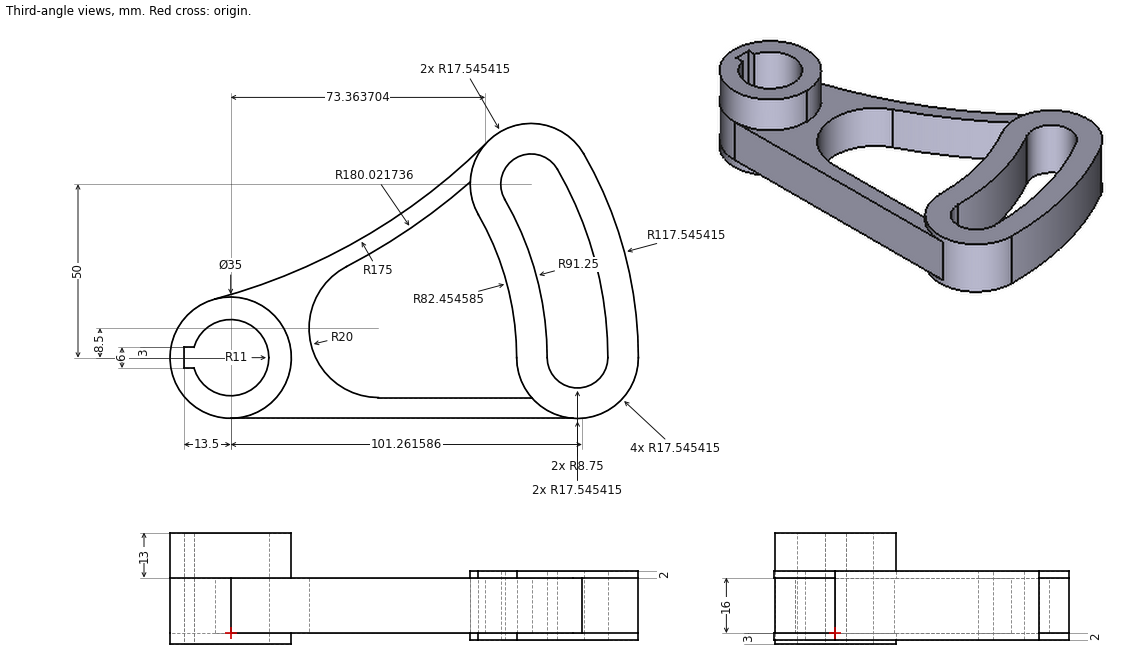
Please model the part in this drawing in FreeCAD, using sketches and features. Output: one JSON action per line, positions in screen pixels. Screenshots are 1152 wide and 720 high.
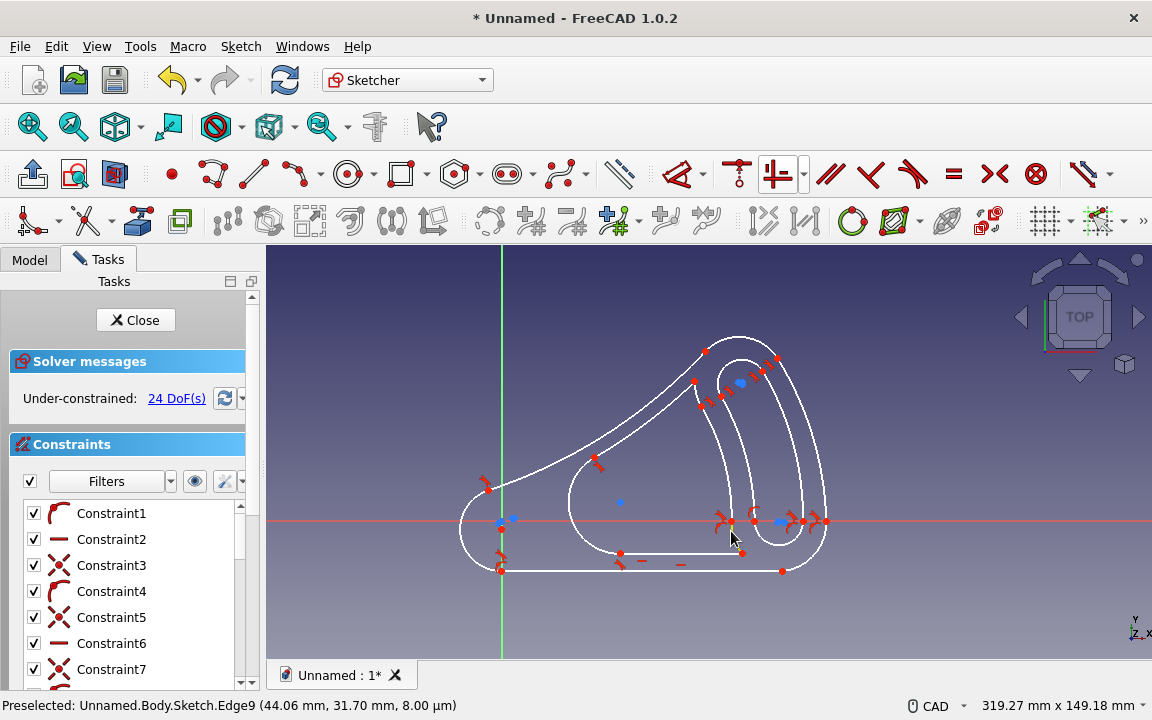
{"action": "left_click", "coordinate": [759, 342]}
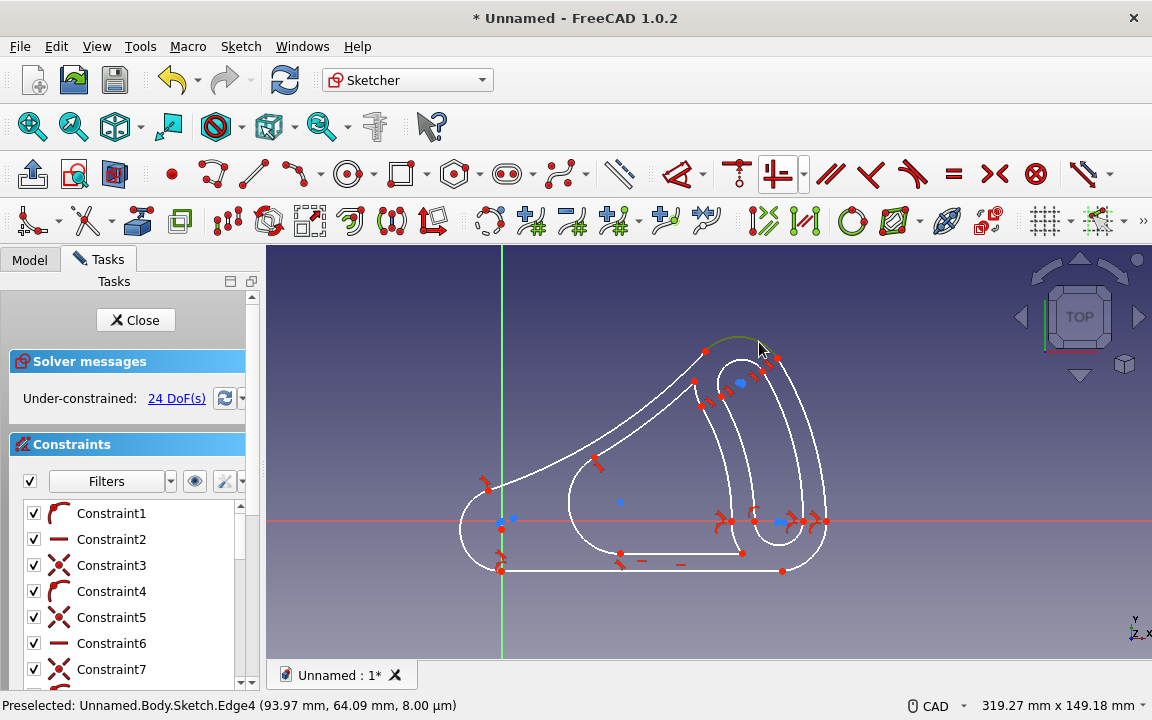
{"action": "scroll", "coordinate": [696, 395], "scroll_direction": "up", "scroll_amount": 2}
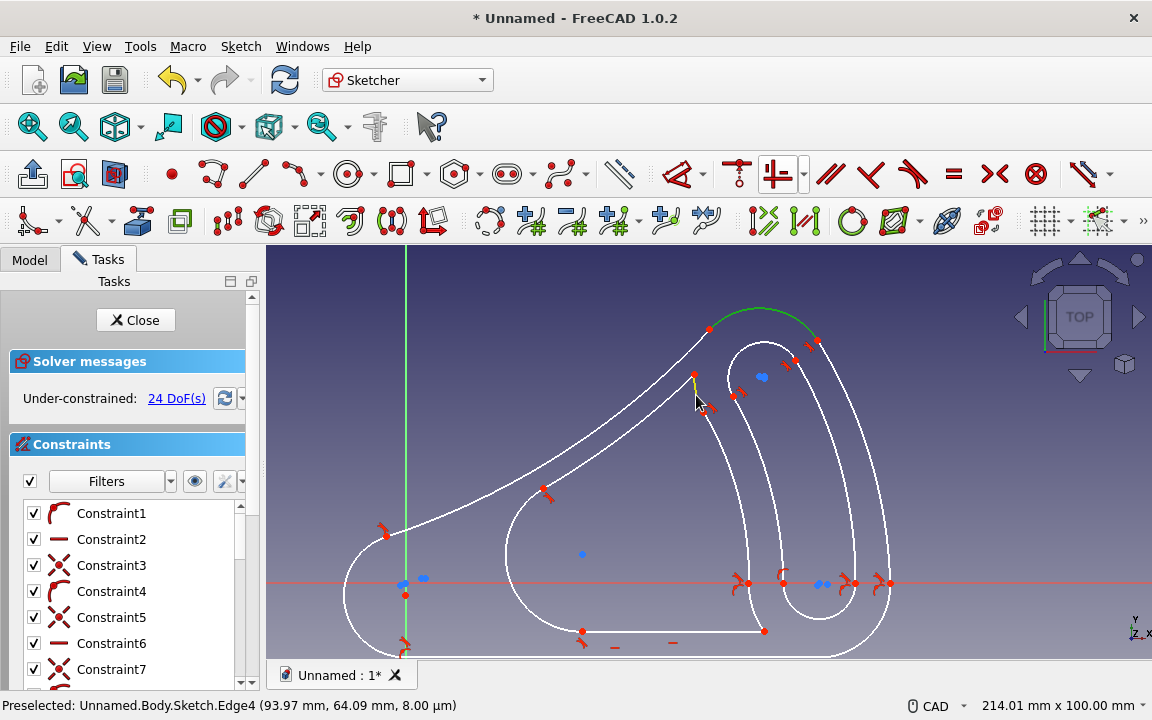
{"action": "left_click", "coordinate": [696, 394]}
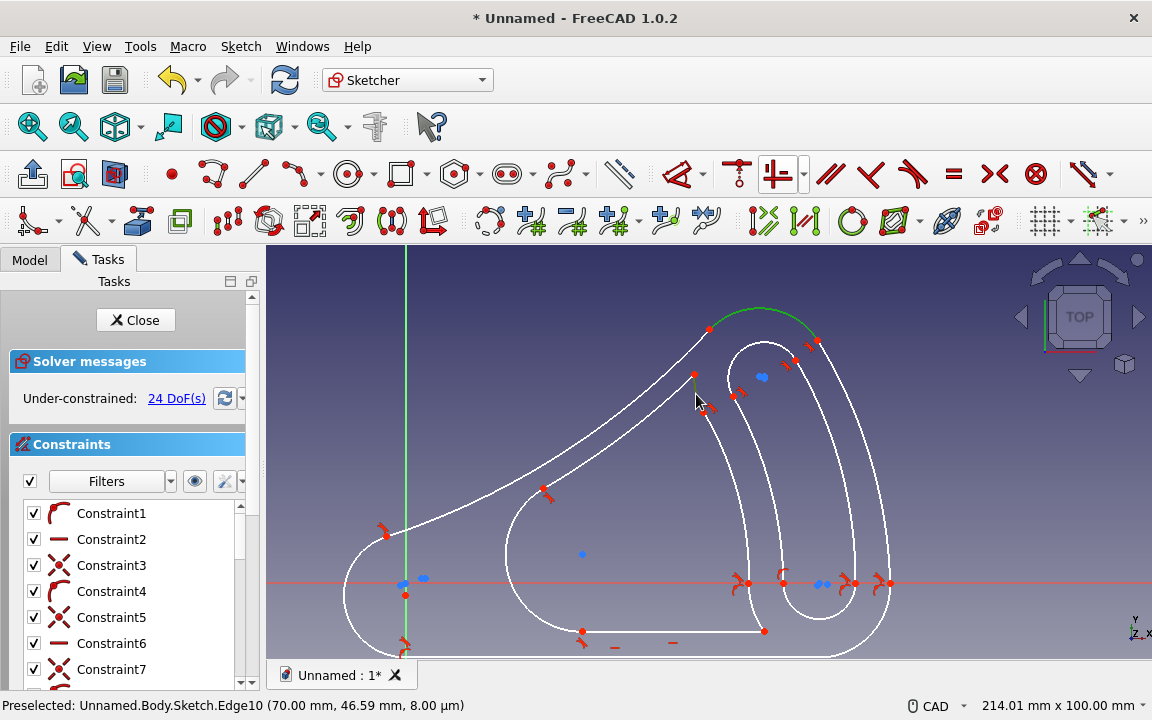
{"action": "left_click", "coordinate": [737, 174]}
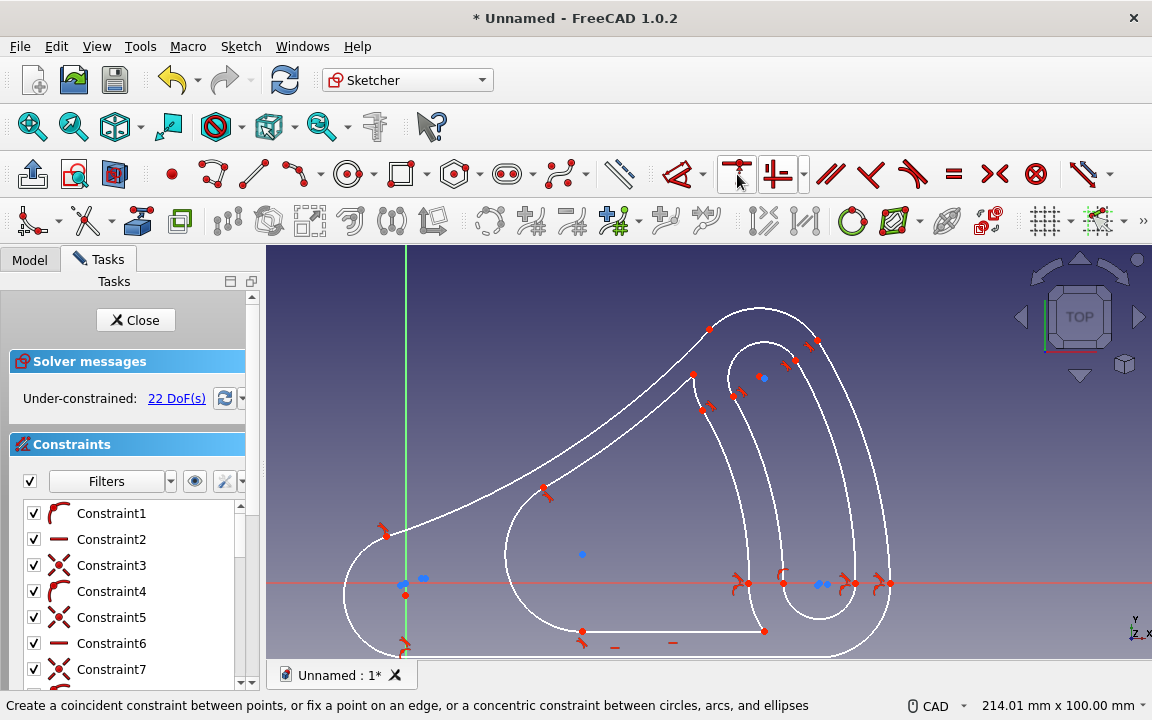
{"action": "left_click", "coordinate": [882, 507]}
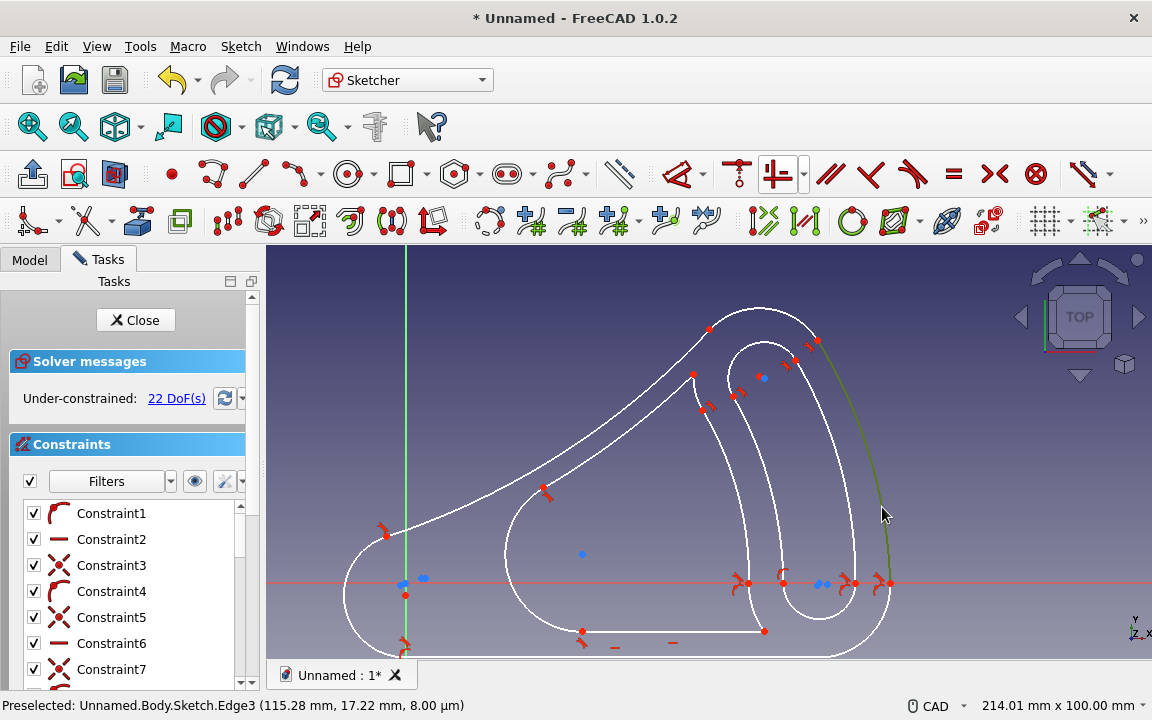
{"action": "left_click", "coordinate": [745, 529]}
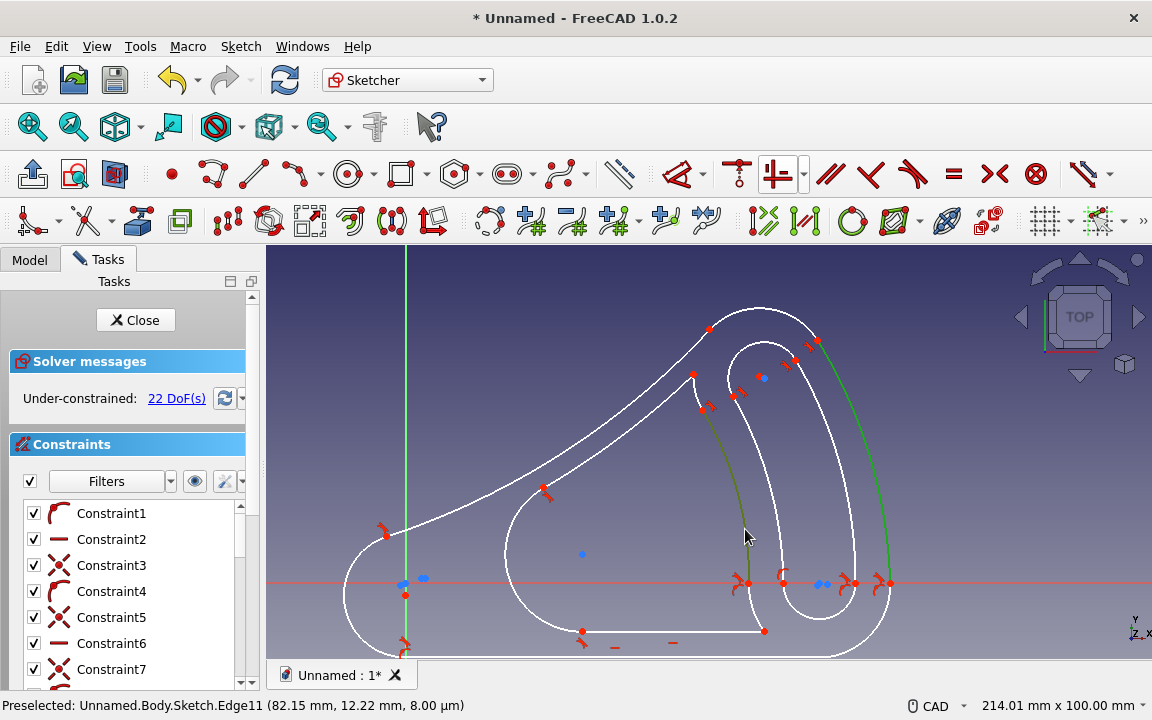
{"action": "left_click", "coordinate": [737, 174]}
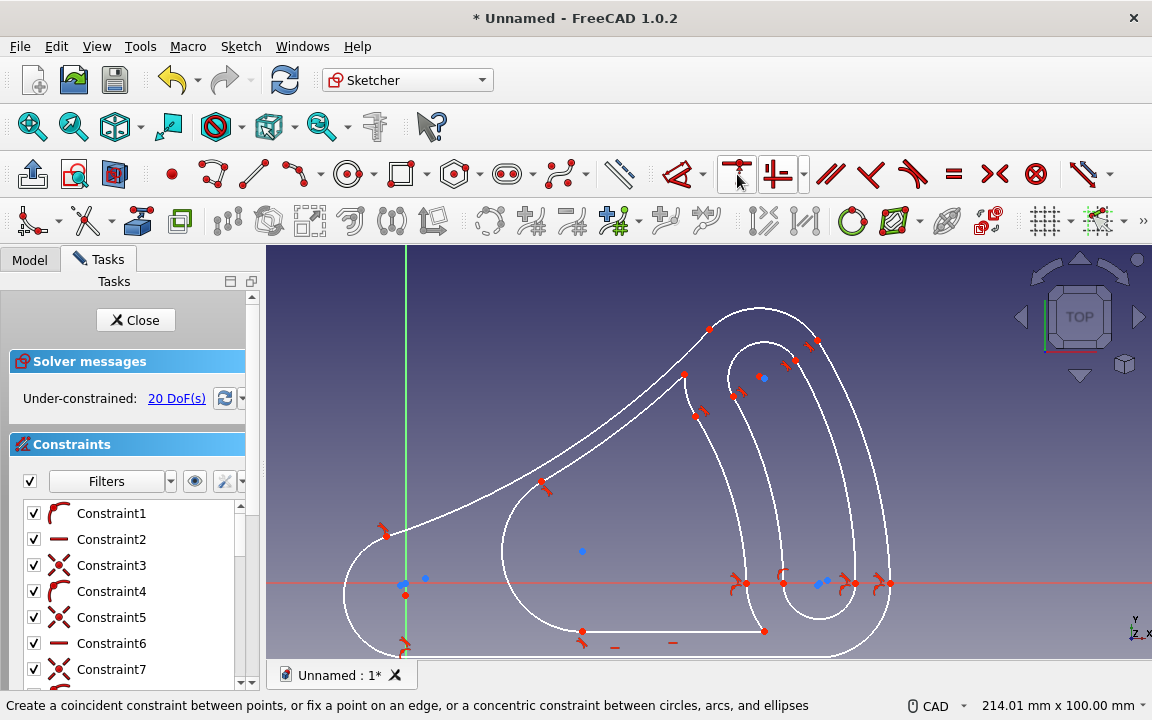
{"action": "left_click", "coordinate": [790, 316]}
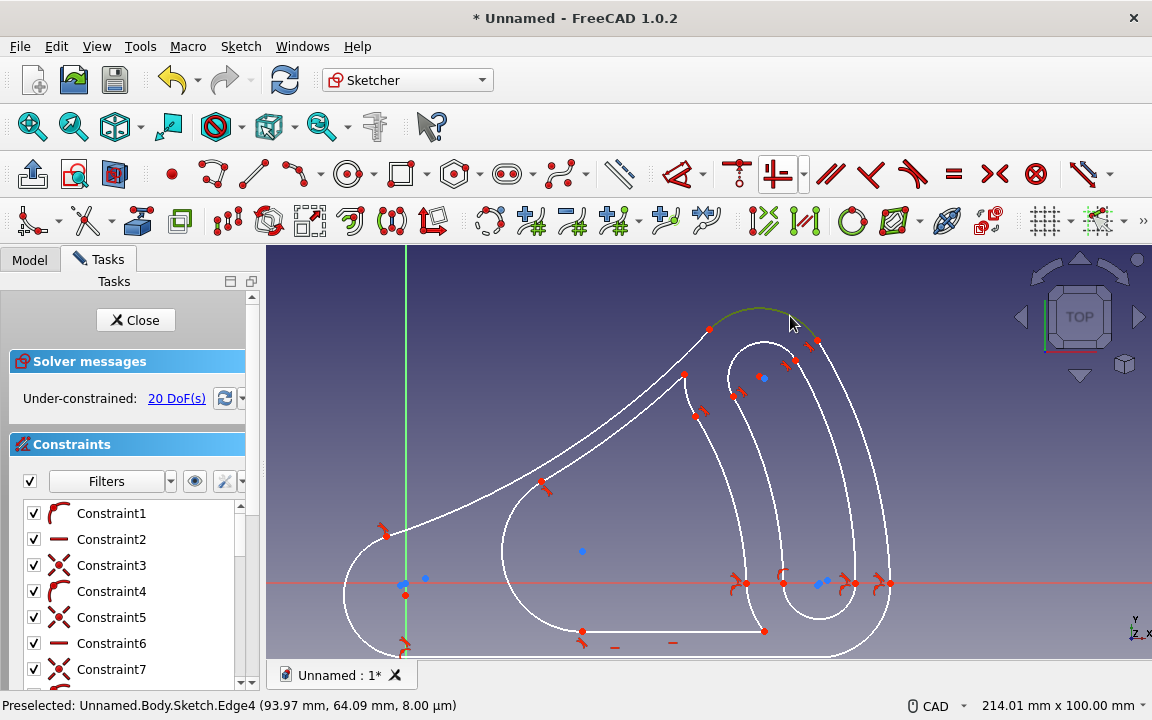
{"action": "left_click", "coordinate": [768, 342]}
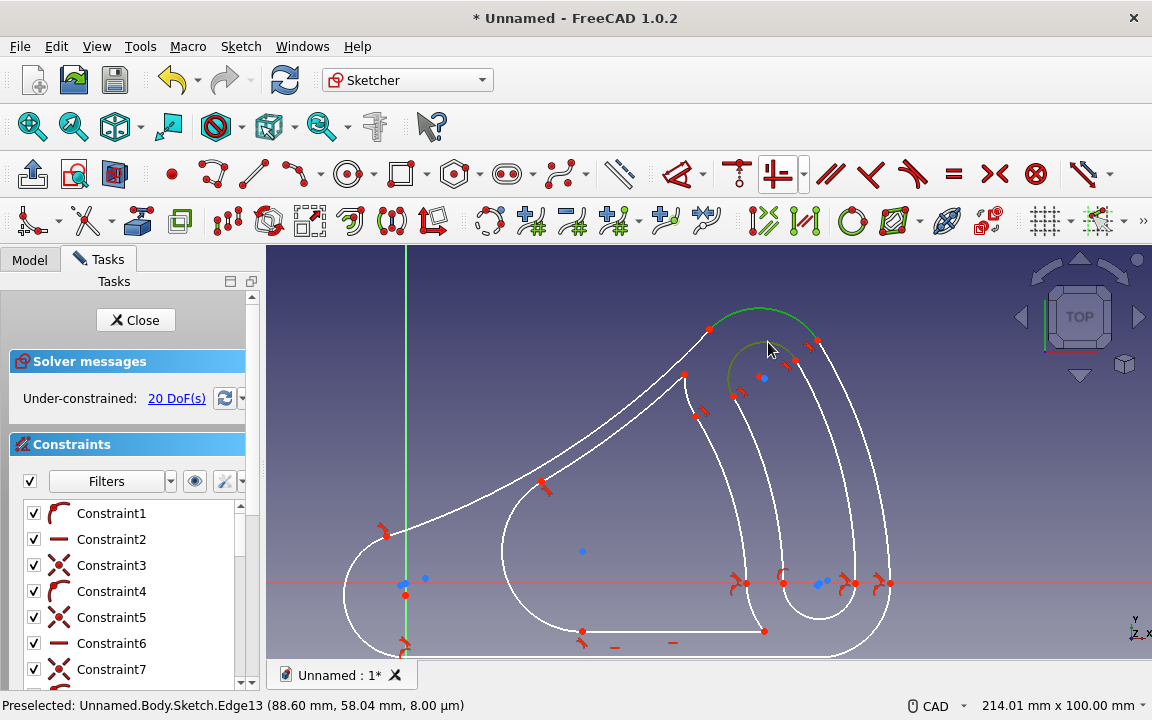
{"action": "left_click", "coordinate": [737, 174]}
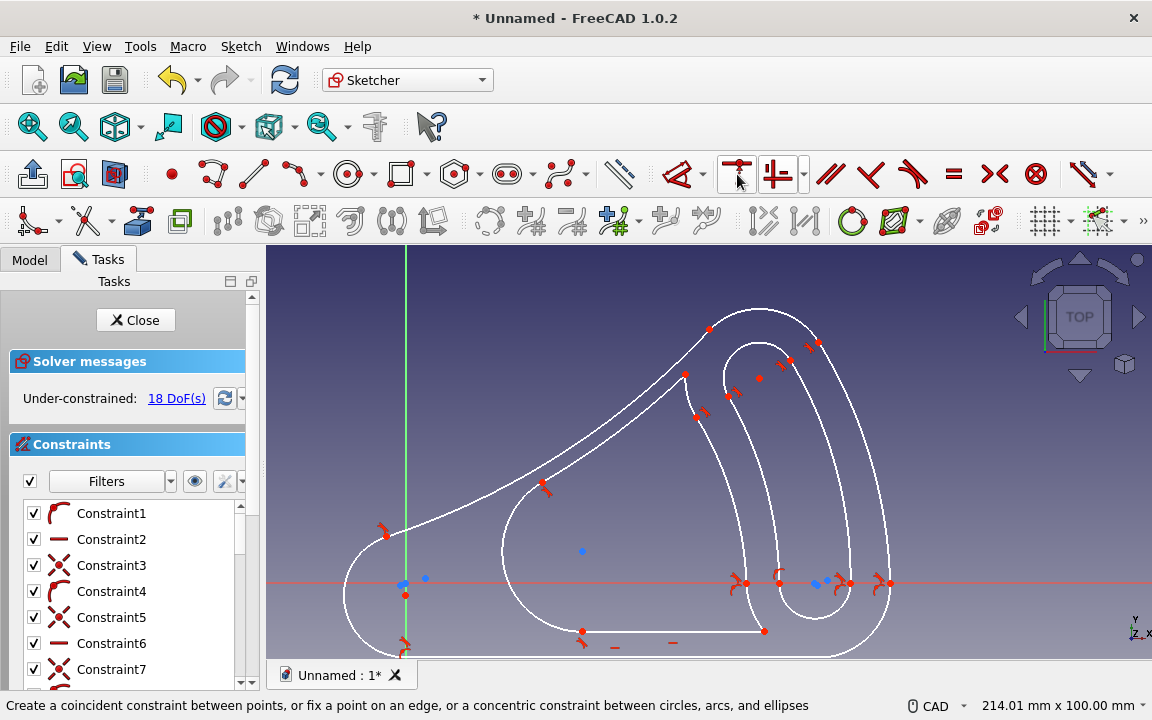
{"action": "left_click", "coordinate": [882, 508]}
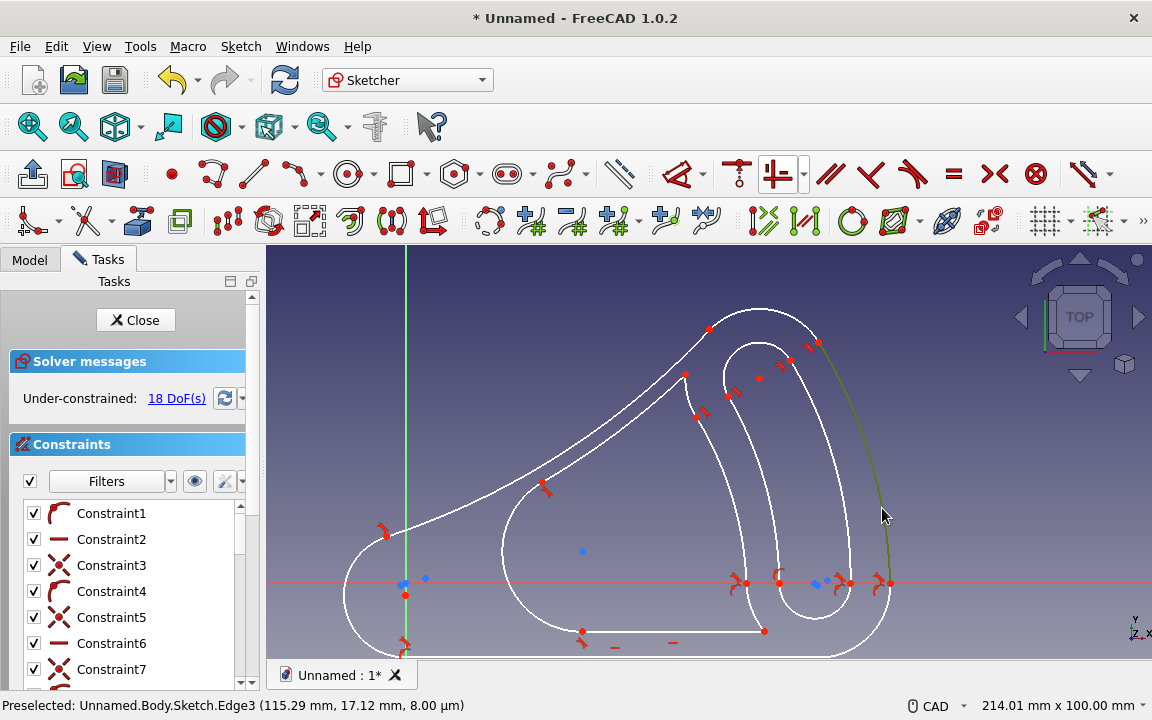
{"action": "left_click", "coordinate": [846, 513]}